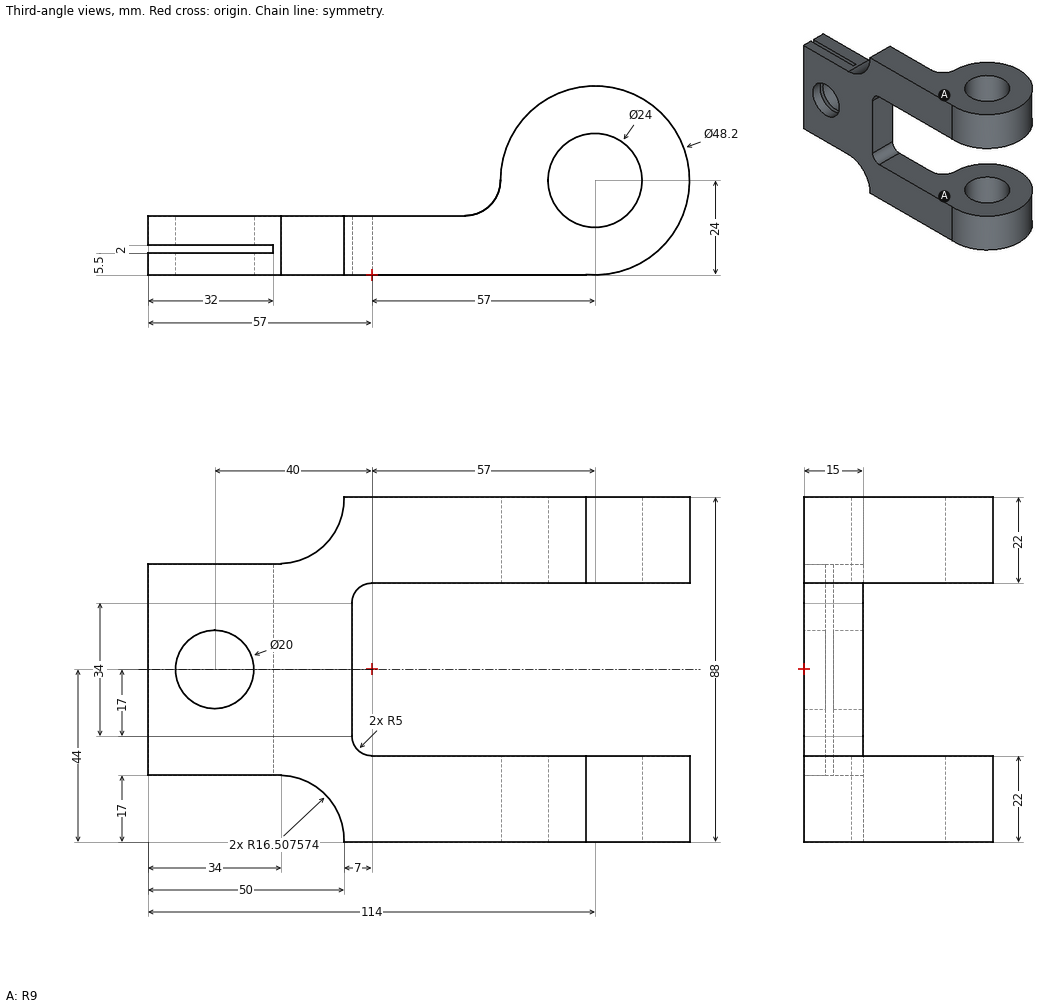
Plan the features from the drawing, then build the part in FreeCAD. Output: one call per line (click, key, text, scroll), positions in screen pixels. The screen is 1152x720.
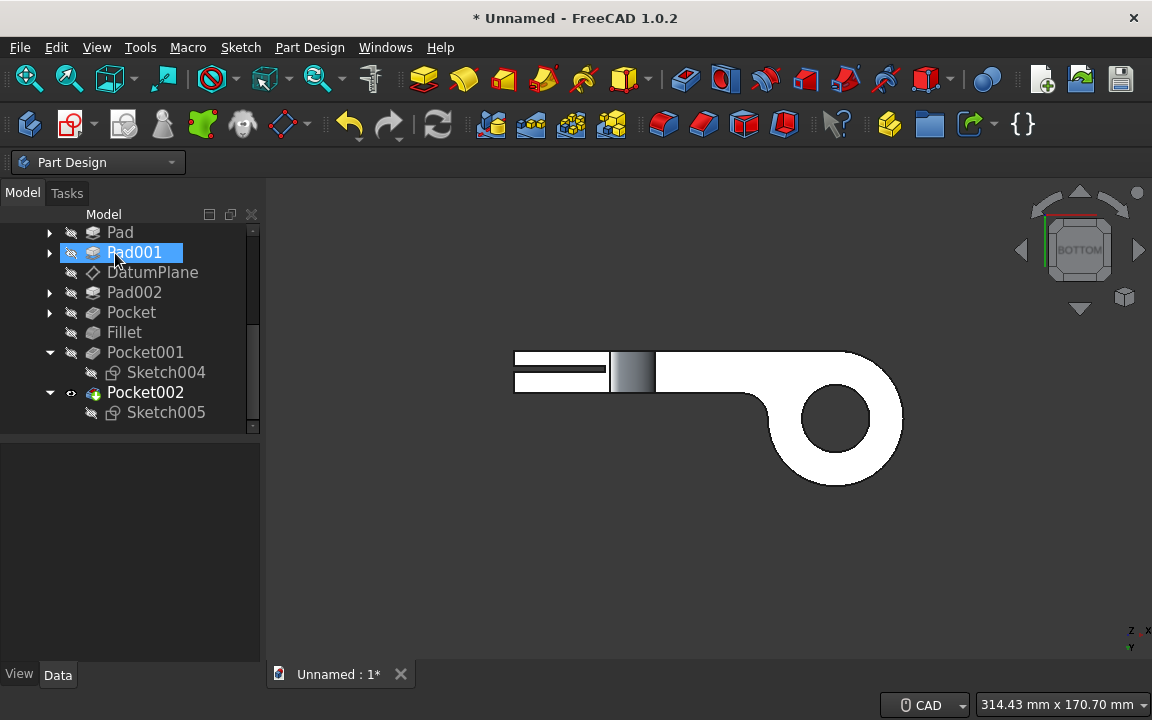
key(0)